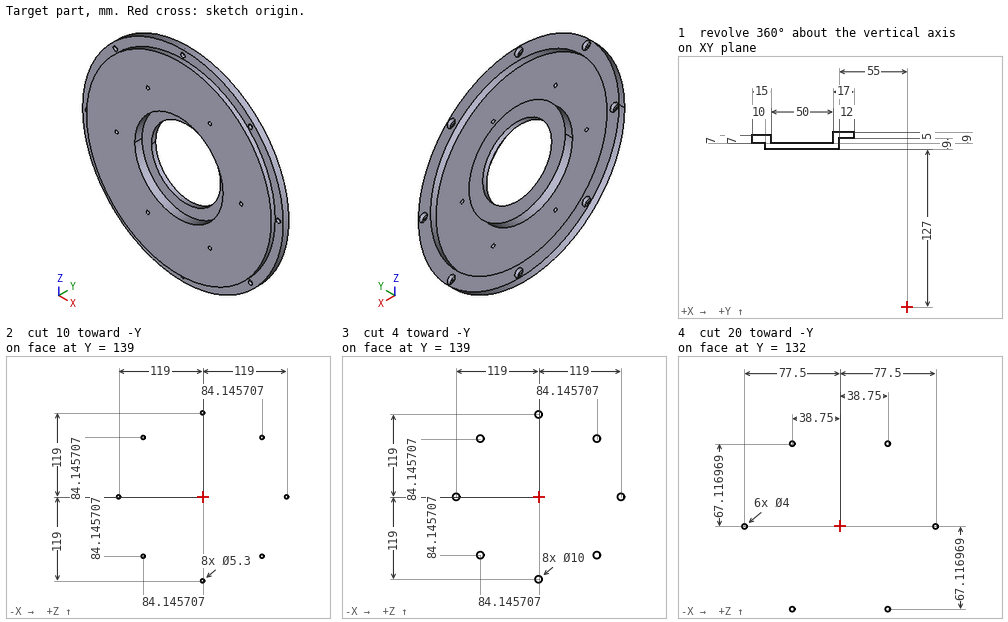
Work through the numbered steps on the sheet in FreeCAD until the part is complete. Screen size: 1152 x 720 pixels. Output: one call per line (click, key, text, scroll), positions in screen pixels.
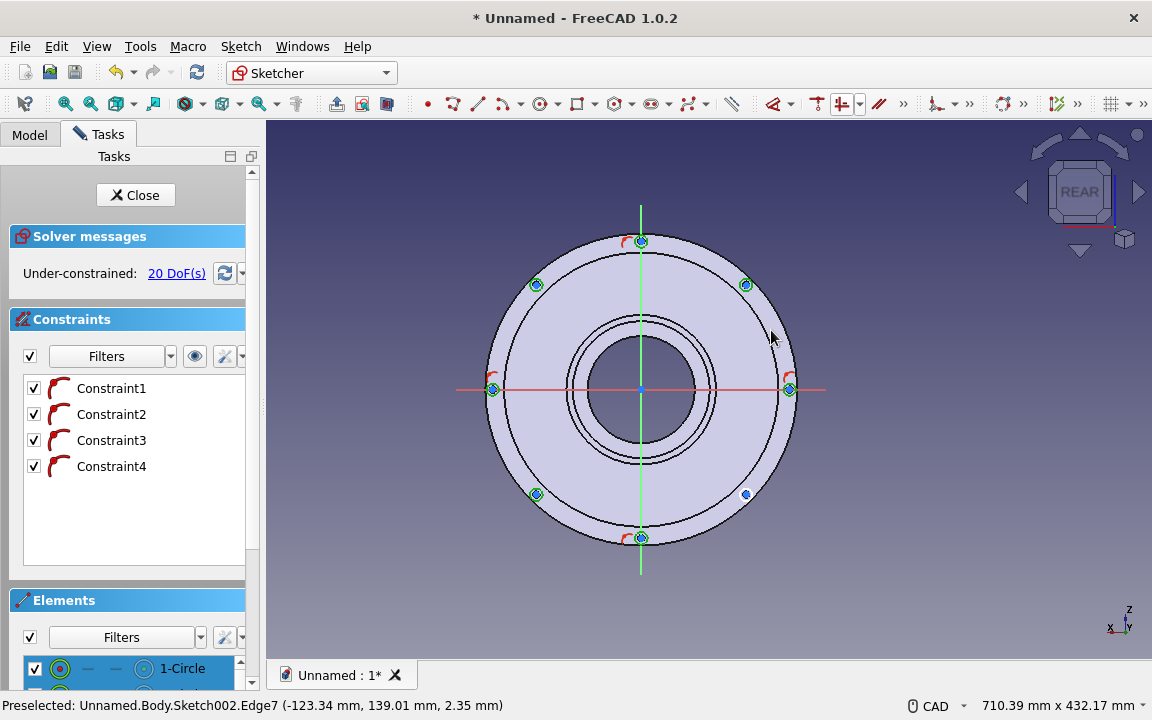
scroll(751, 490, up, 4)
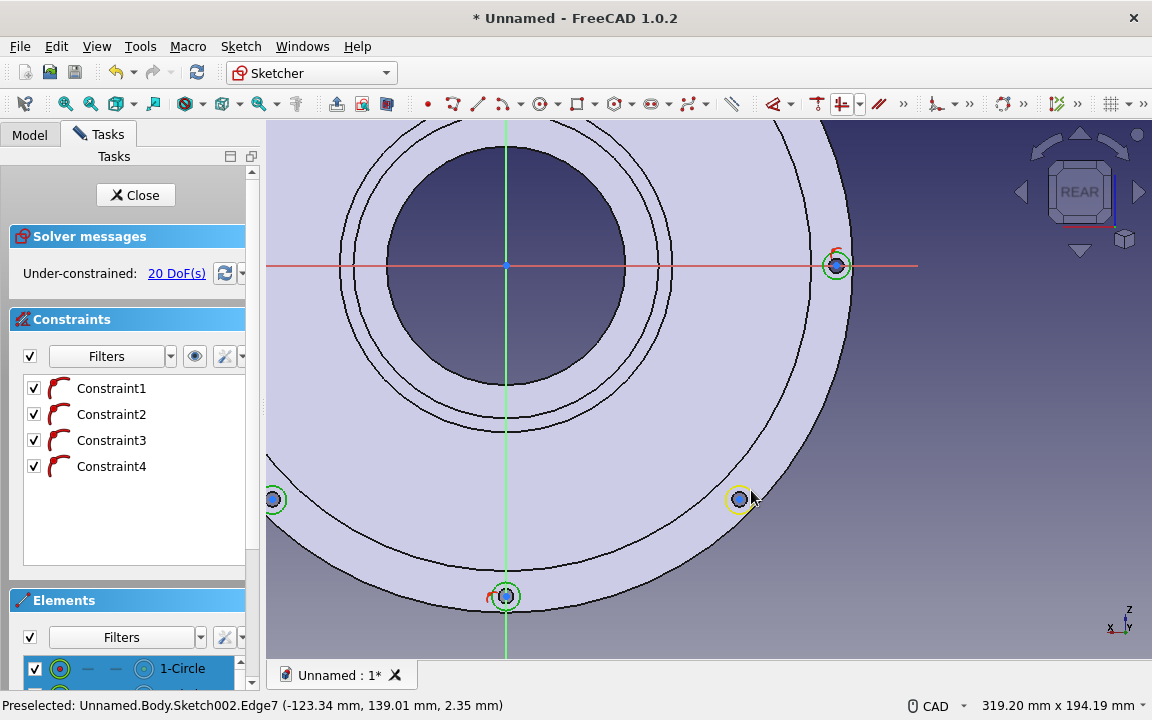
click(749, 490)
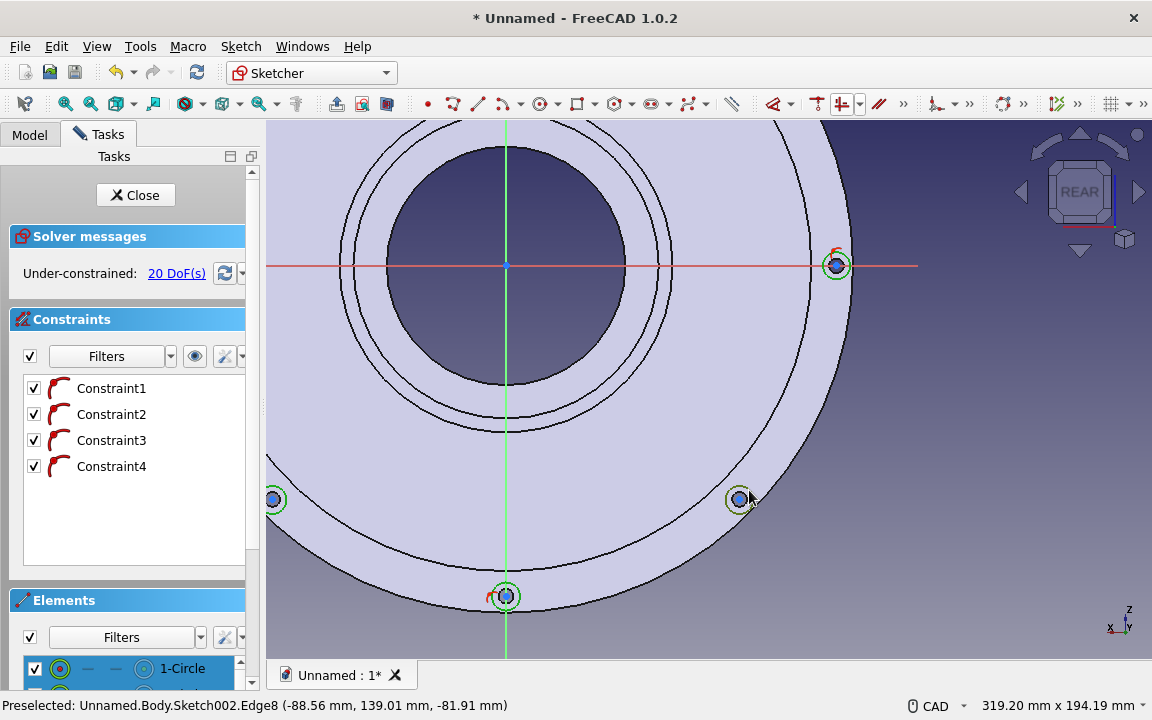
key(e)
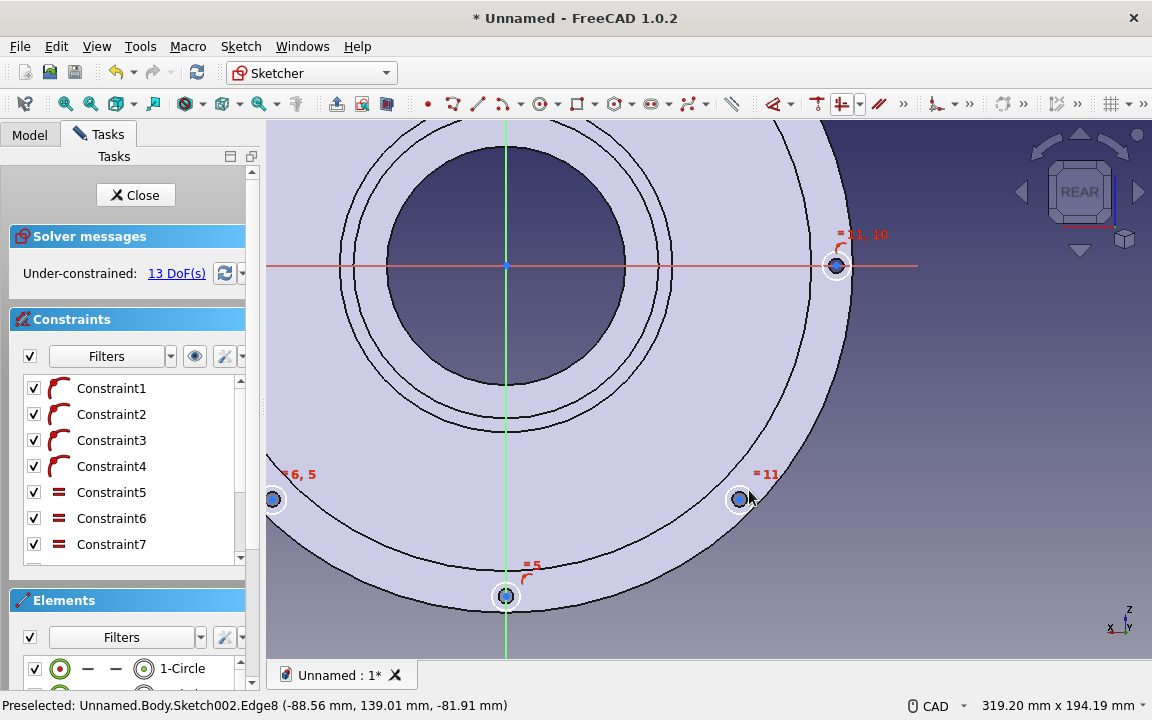
scroll(750, 490, down, 4)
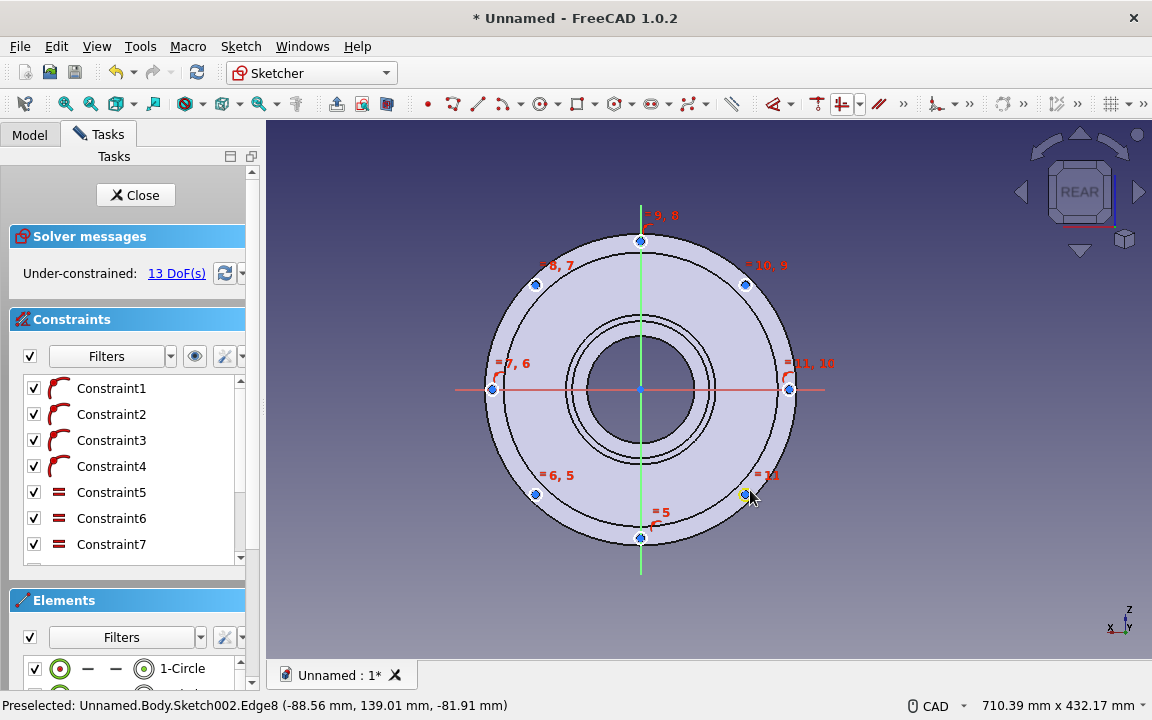
click(536, 495)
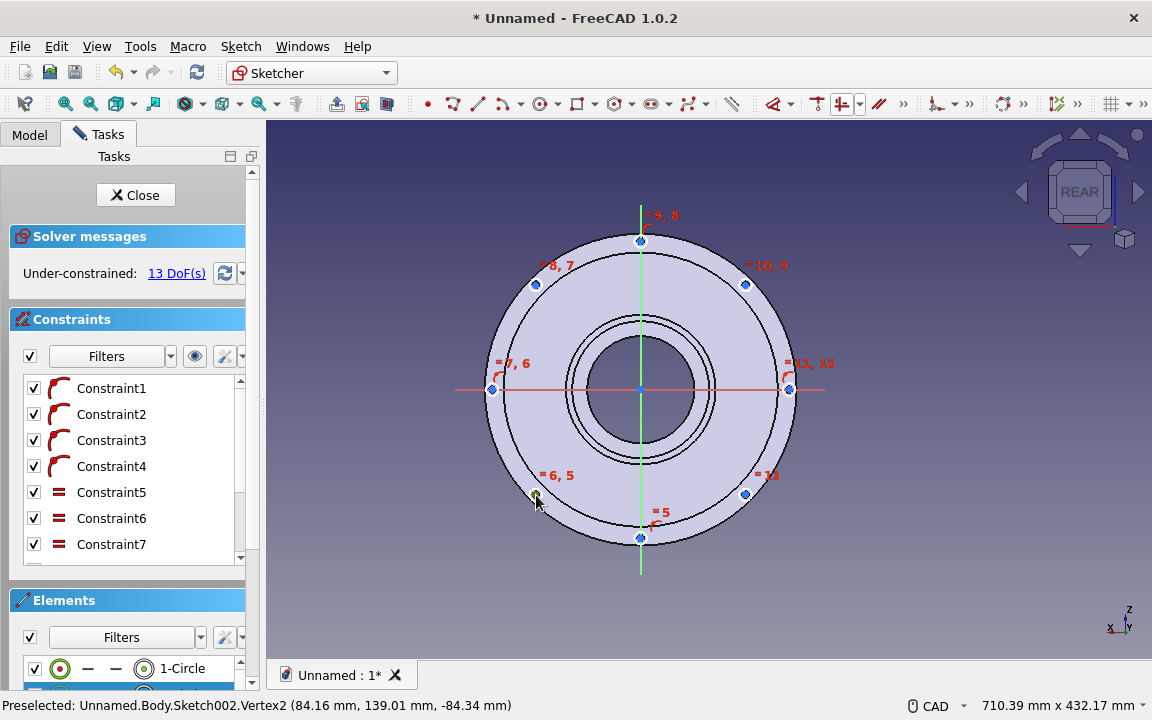
click(536, 285)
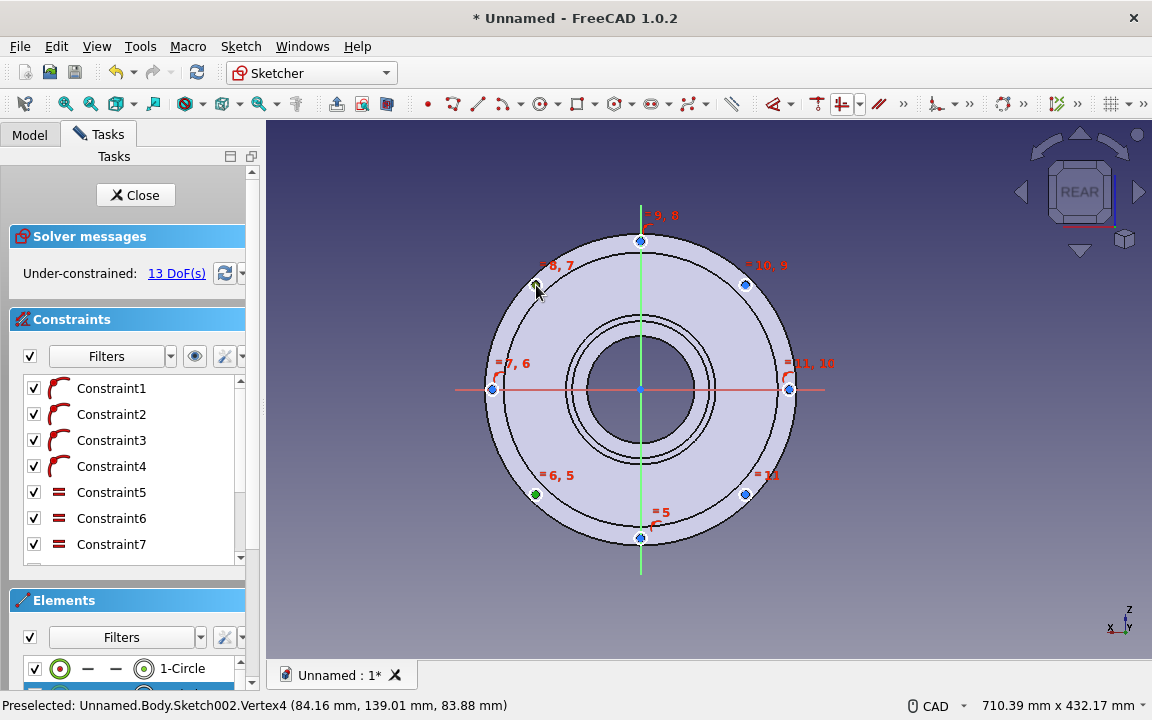
click(860, 104)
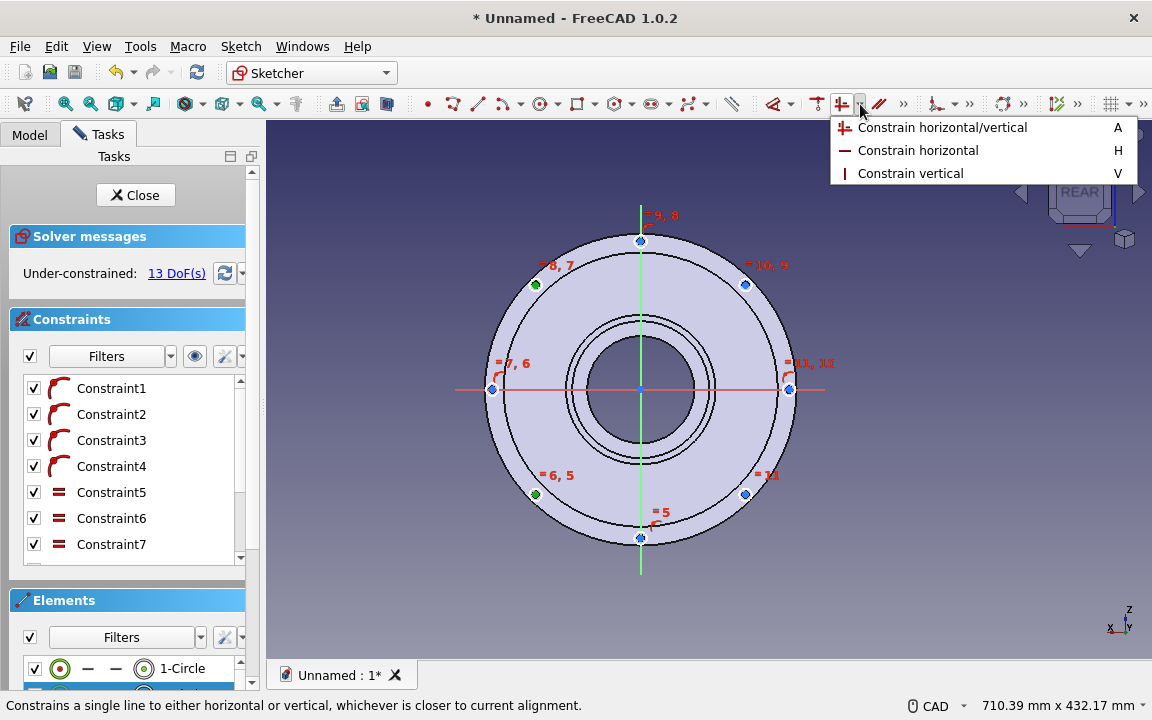
click(984, 174)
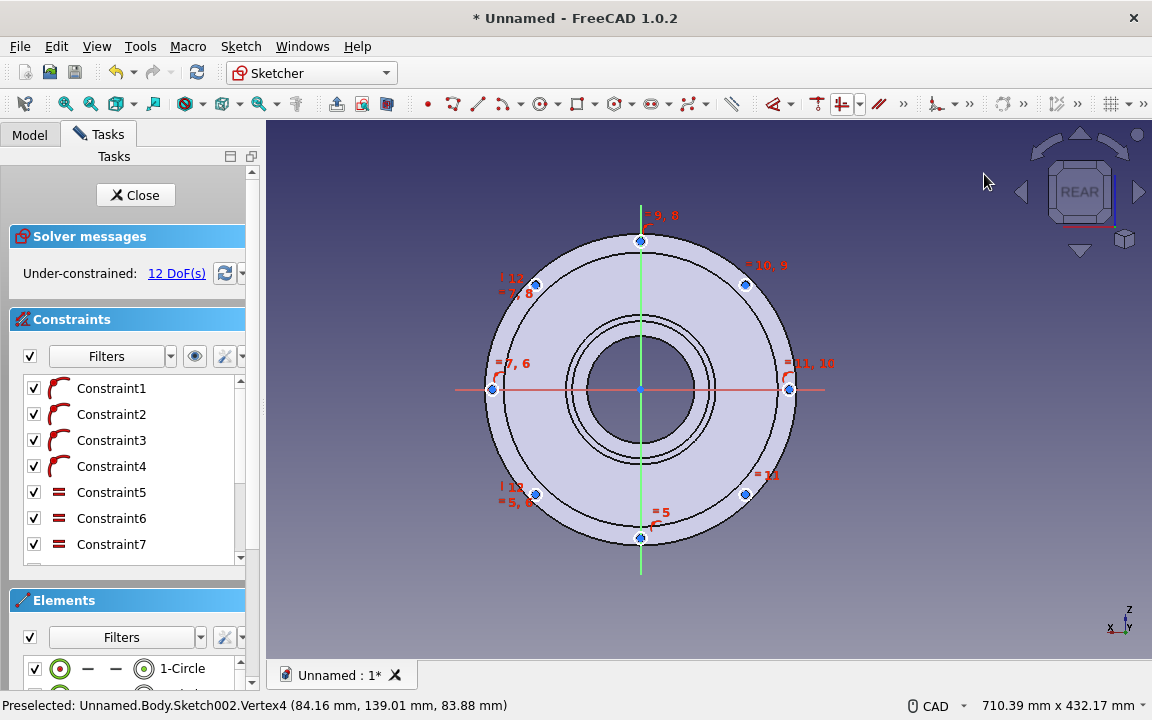
click(536, 285)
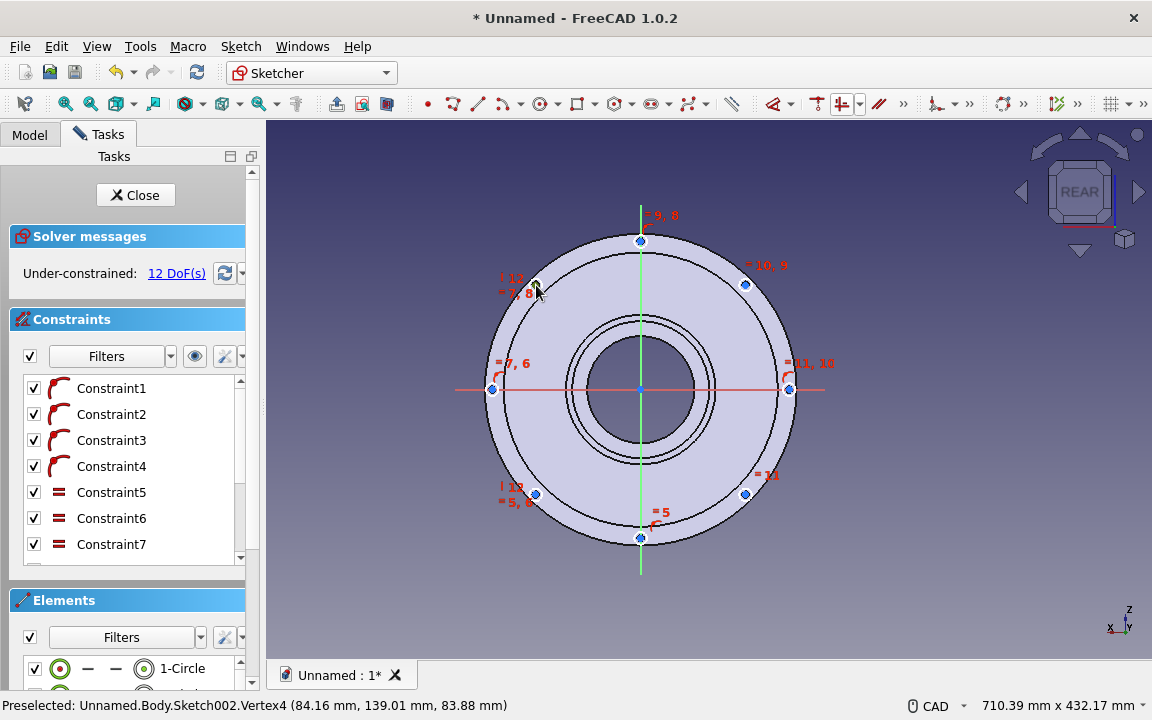
click(746, 285)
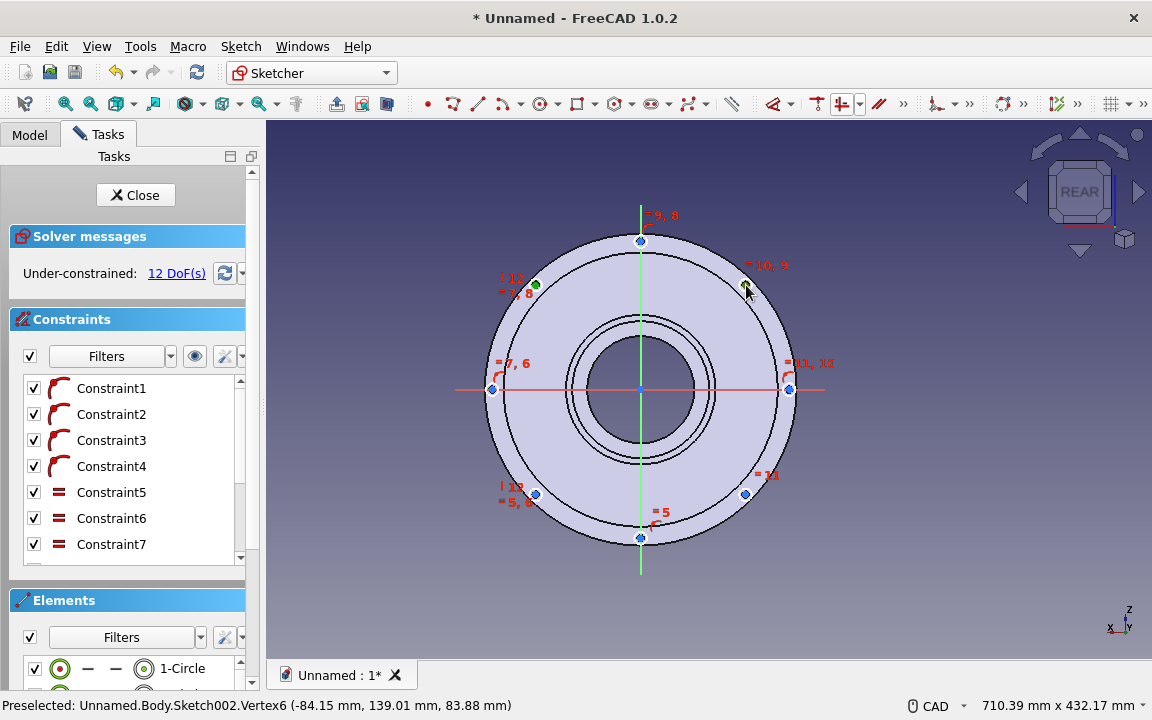
click(860, 104)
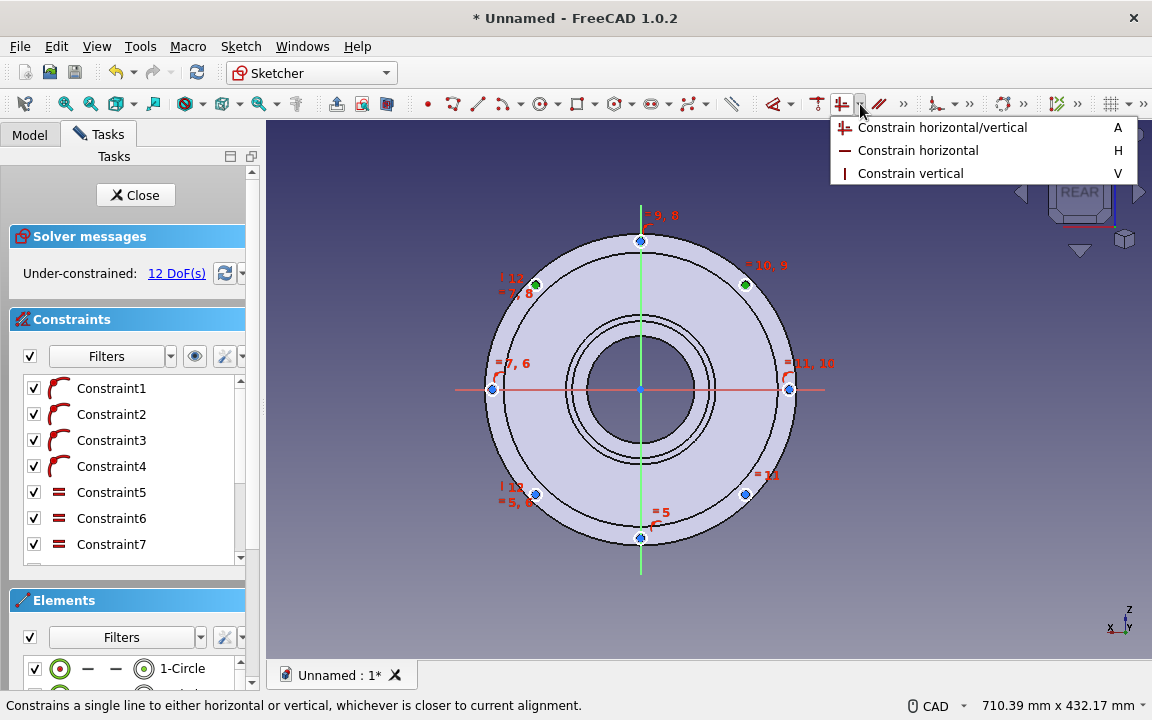
click(984, 150)